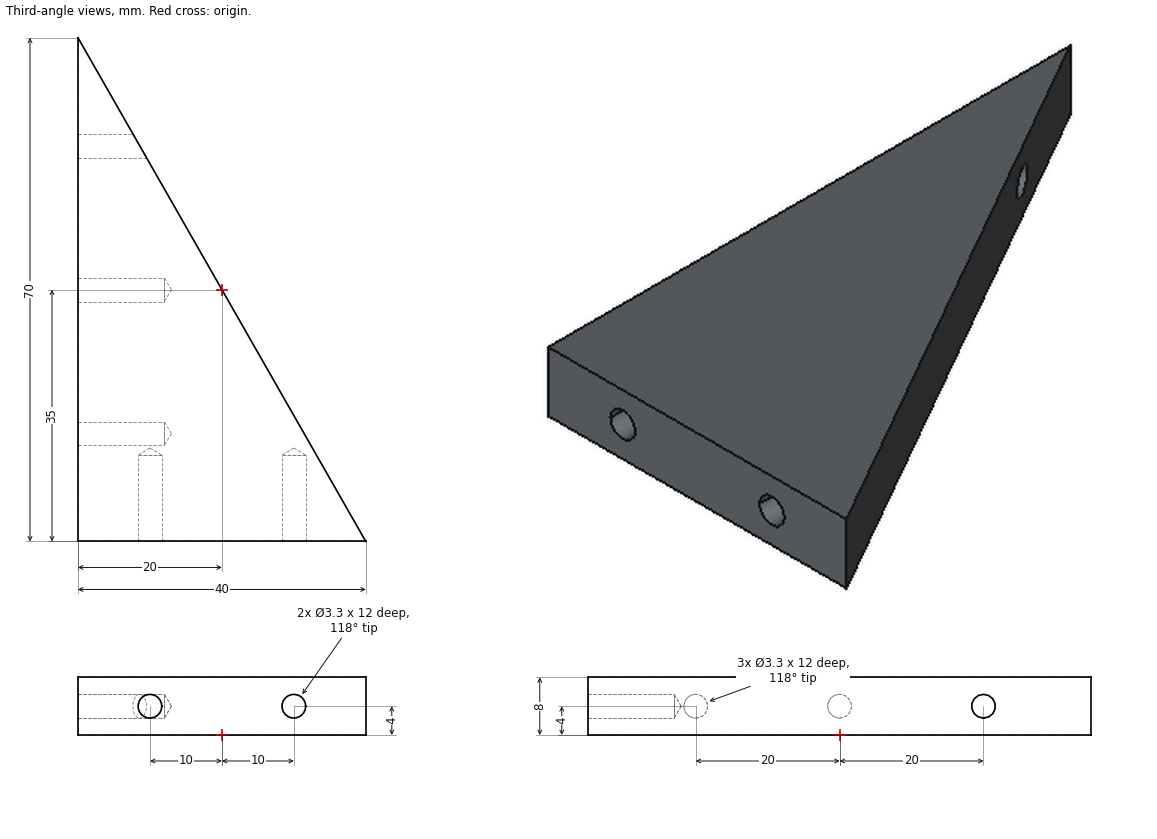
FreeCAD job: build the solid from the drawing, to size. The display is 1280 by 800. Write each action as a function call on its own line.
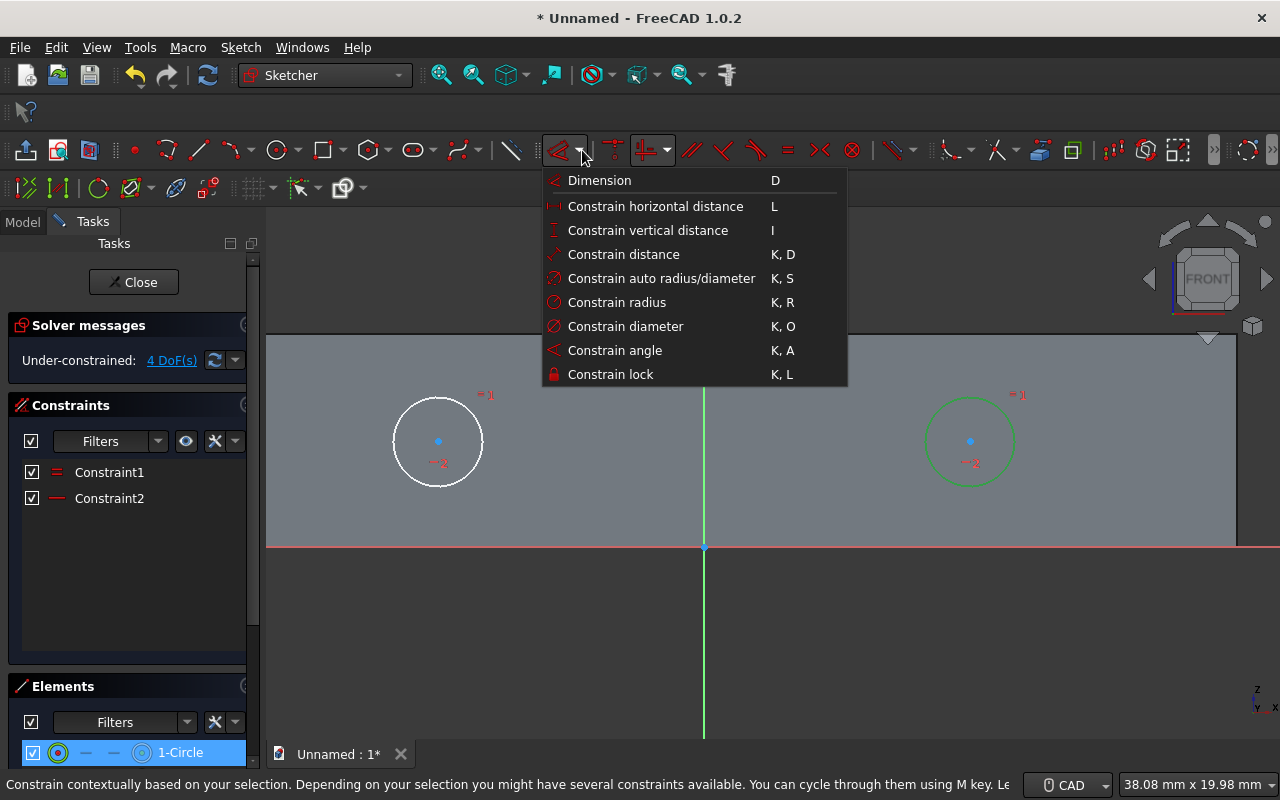
click(695, 326)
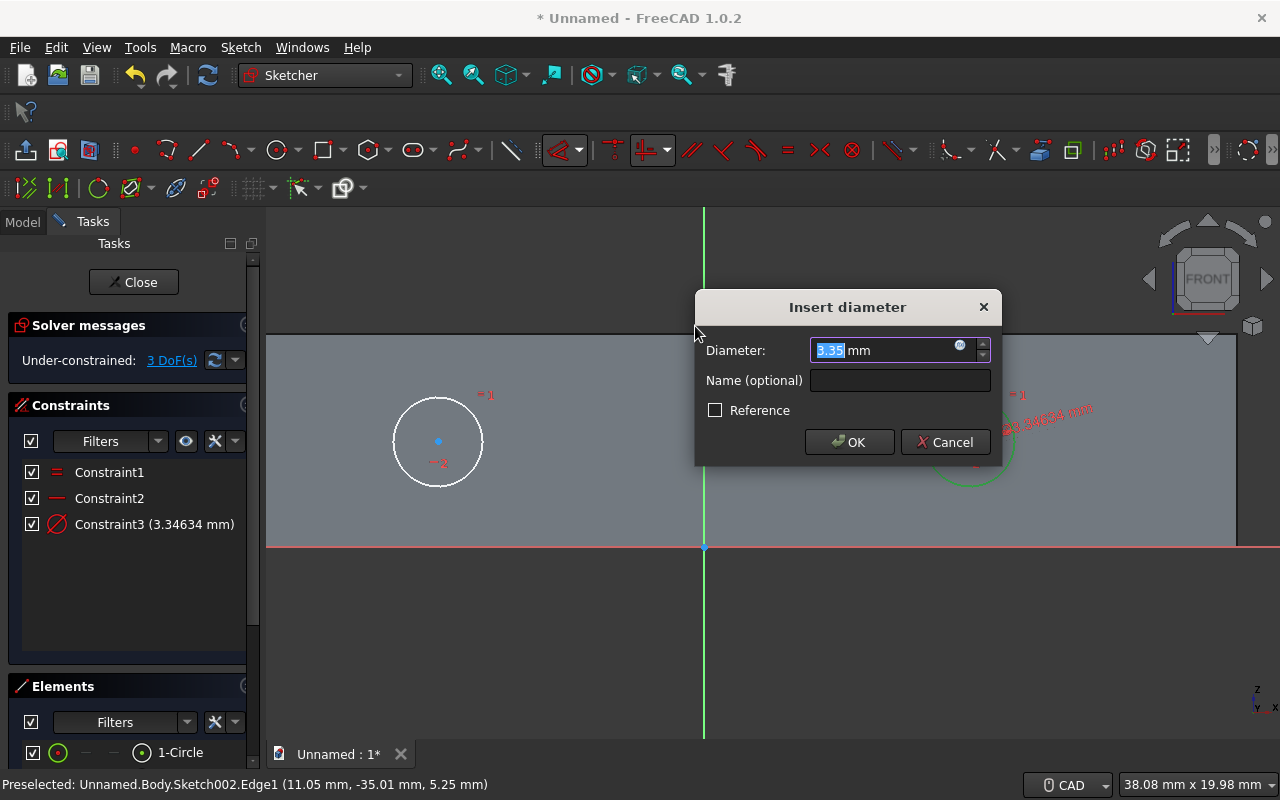
text(3.3)
key(Return)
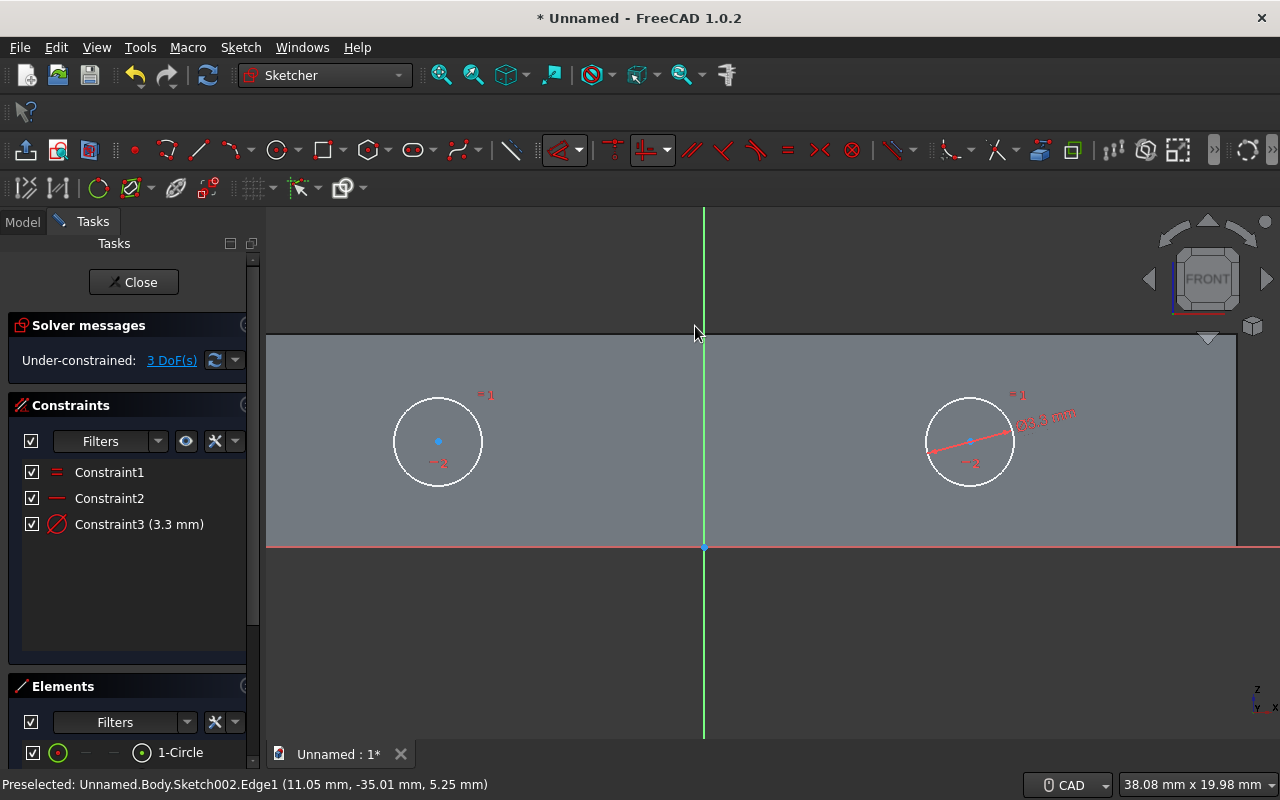
click(970, 442)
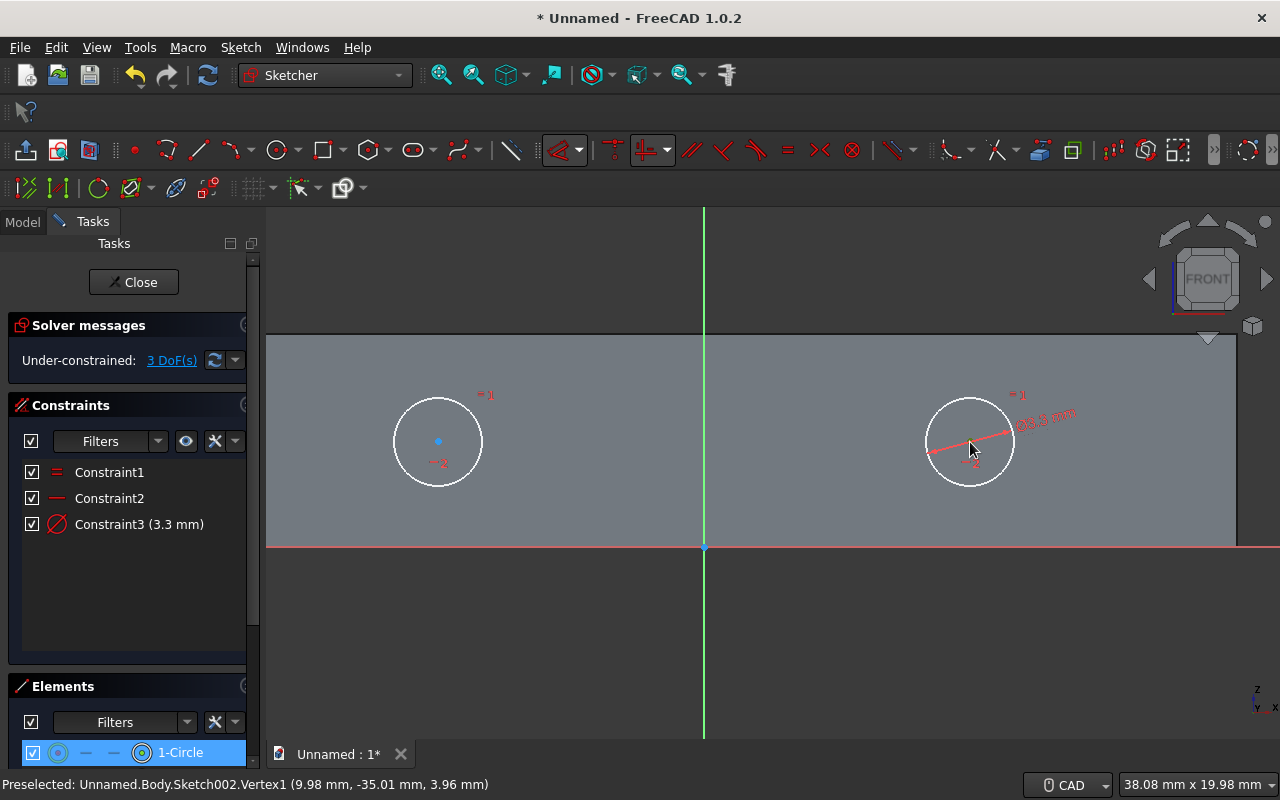
click(582, 150)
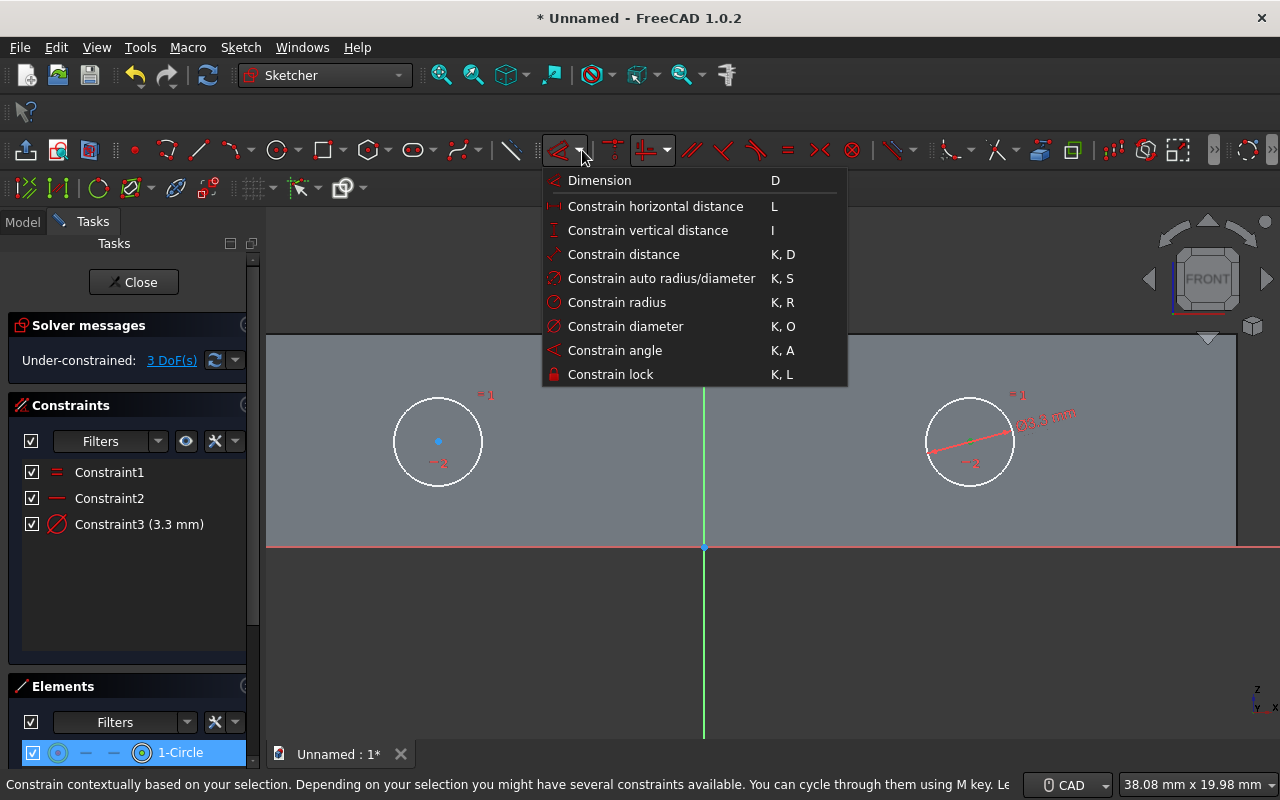
click(695, 230)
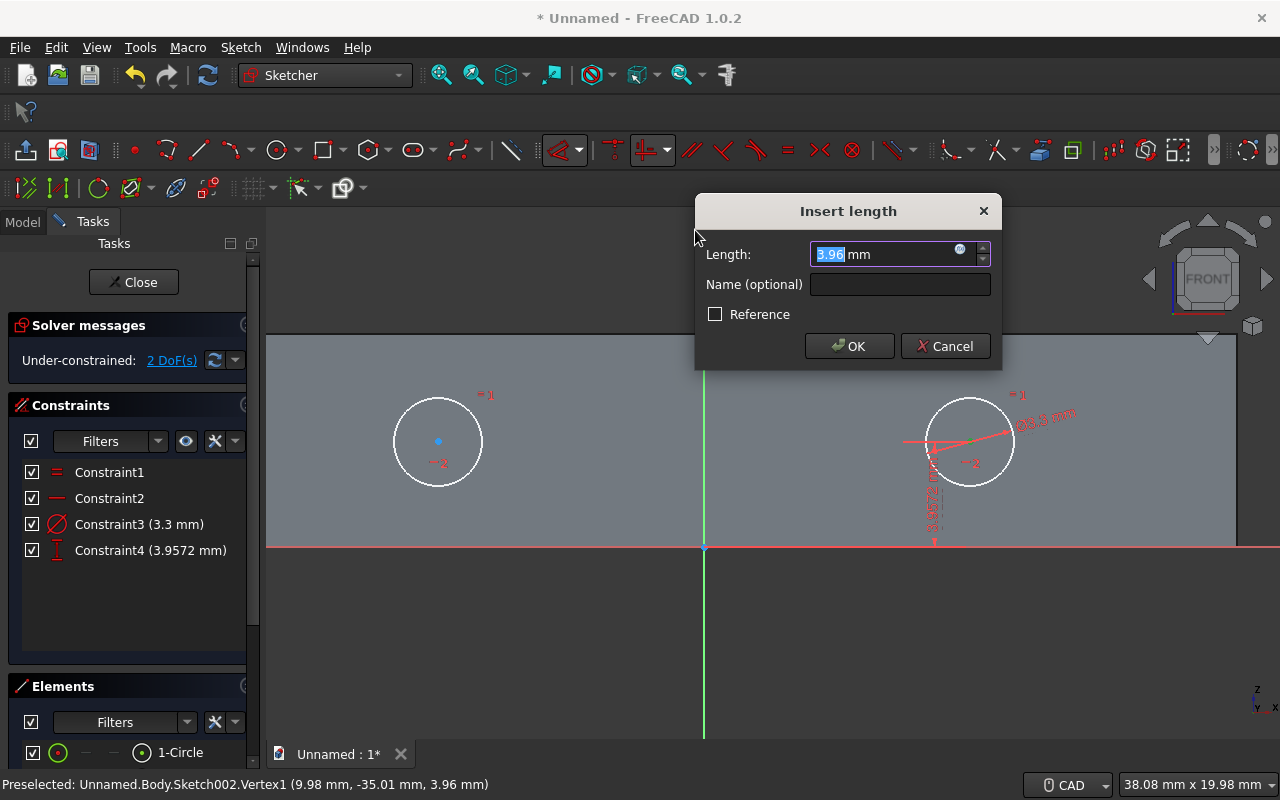
text(4)
key(Return)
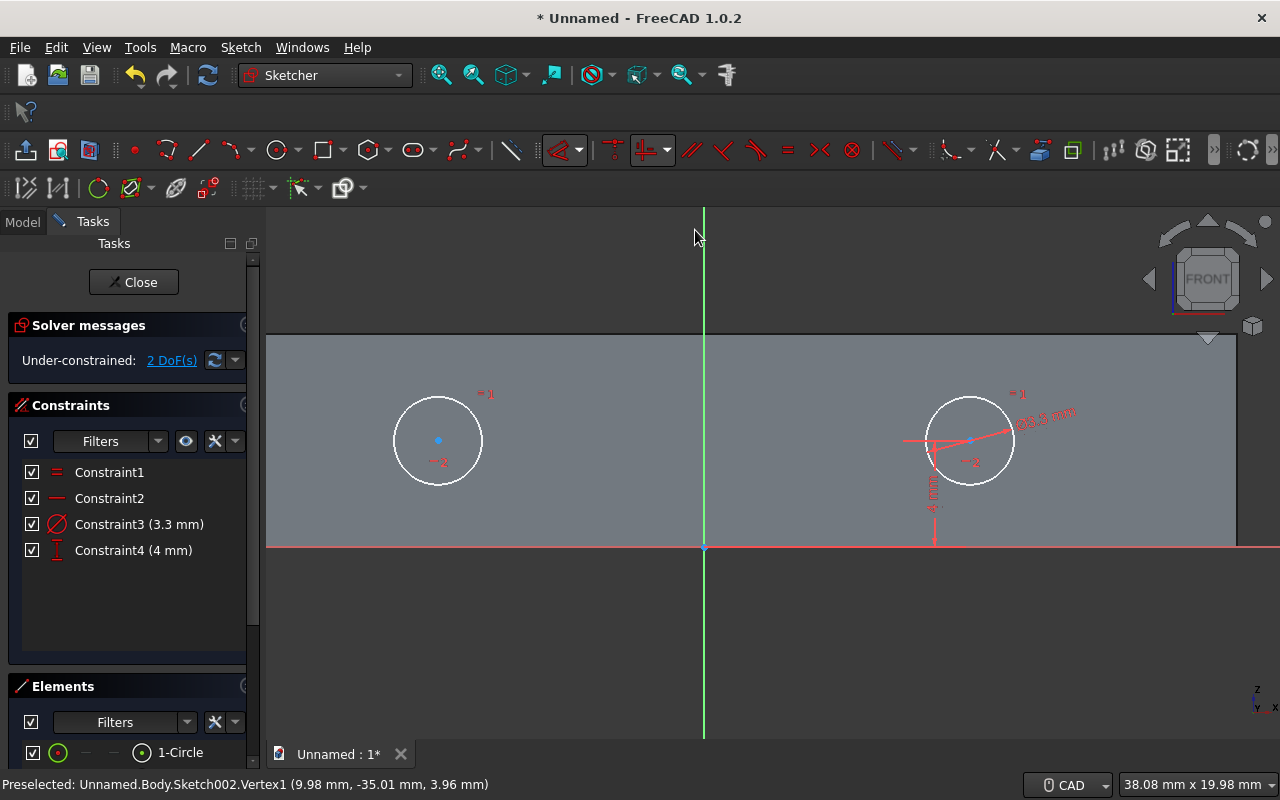
click(970, 441)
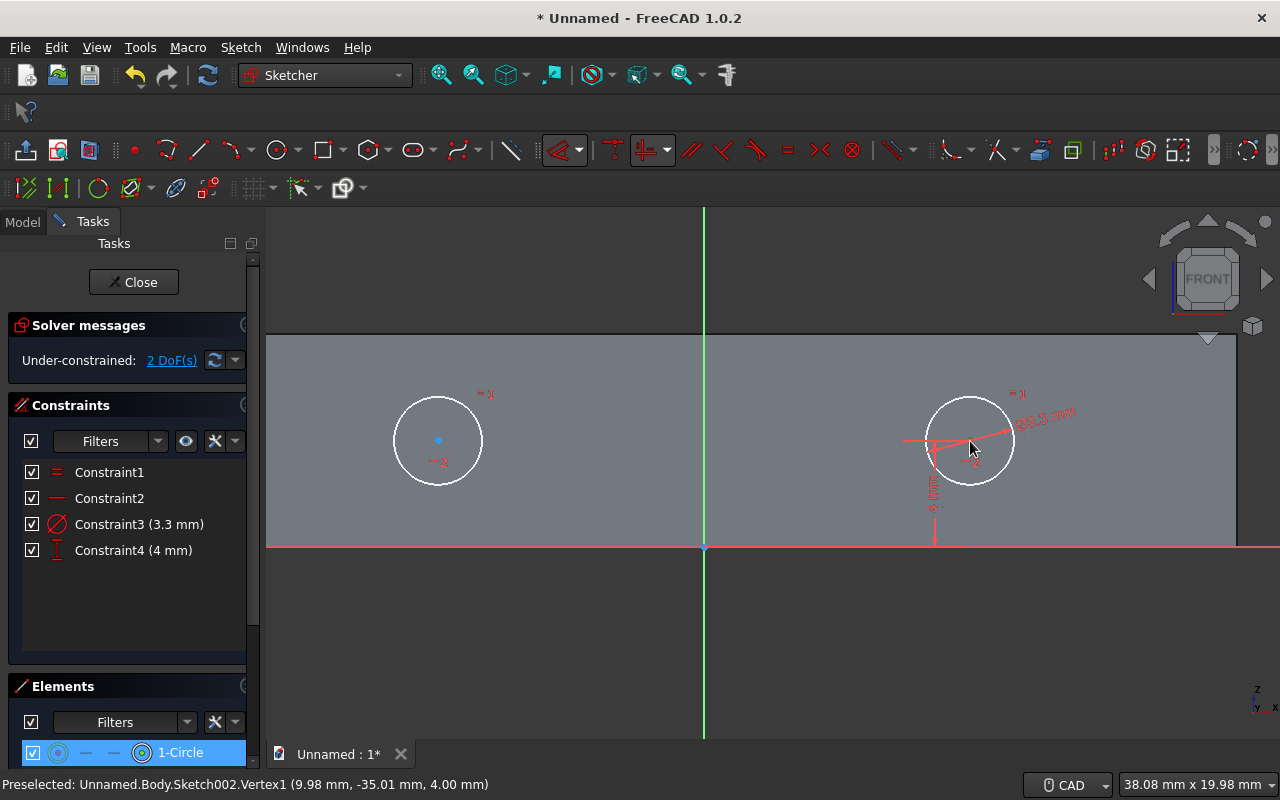
key(l)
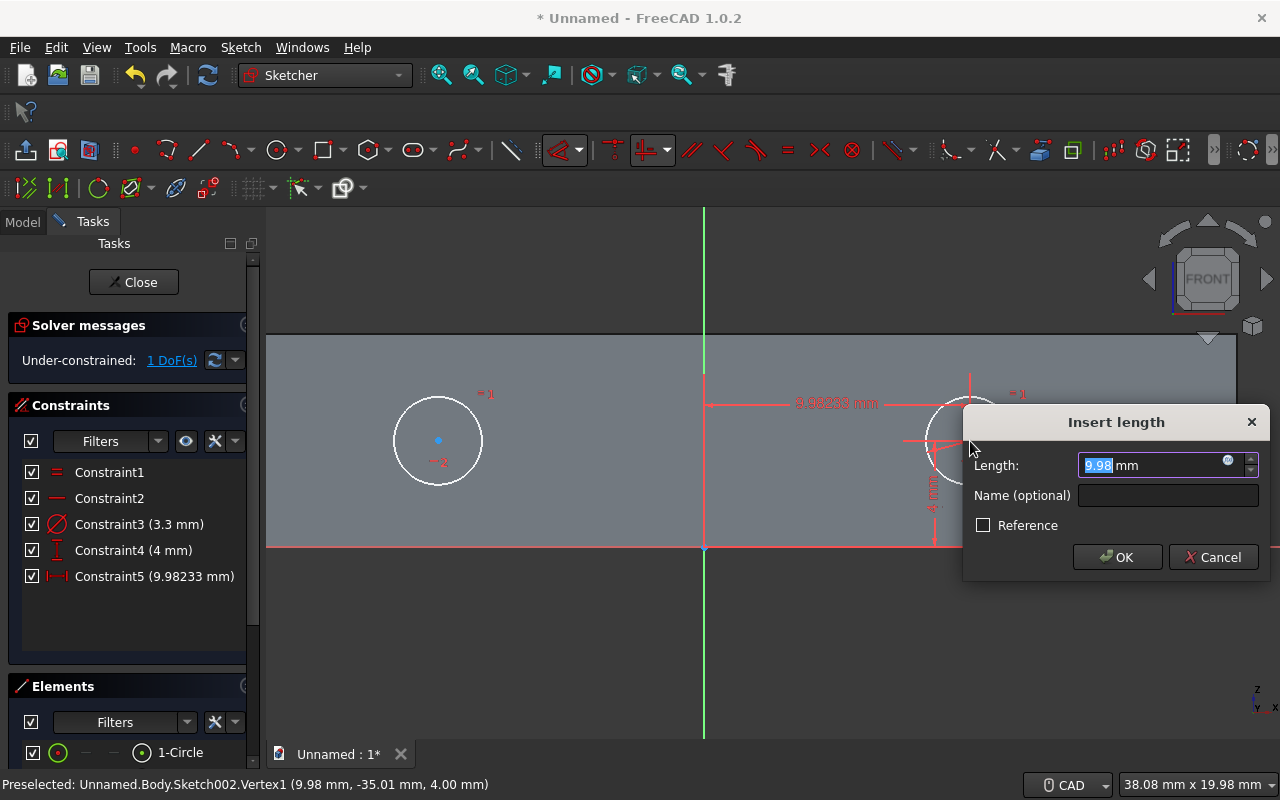
text(10)
key(Return)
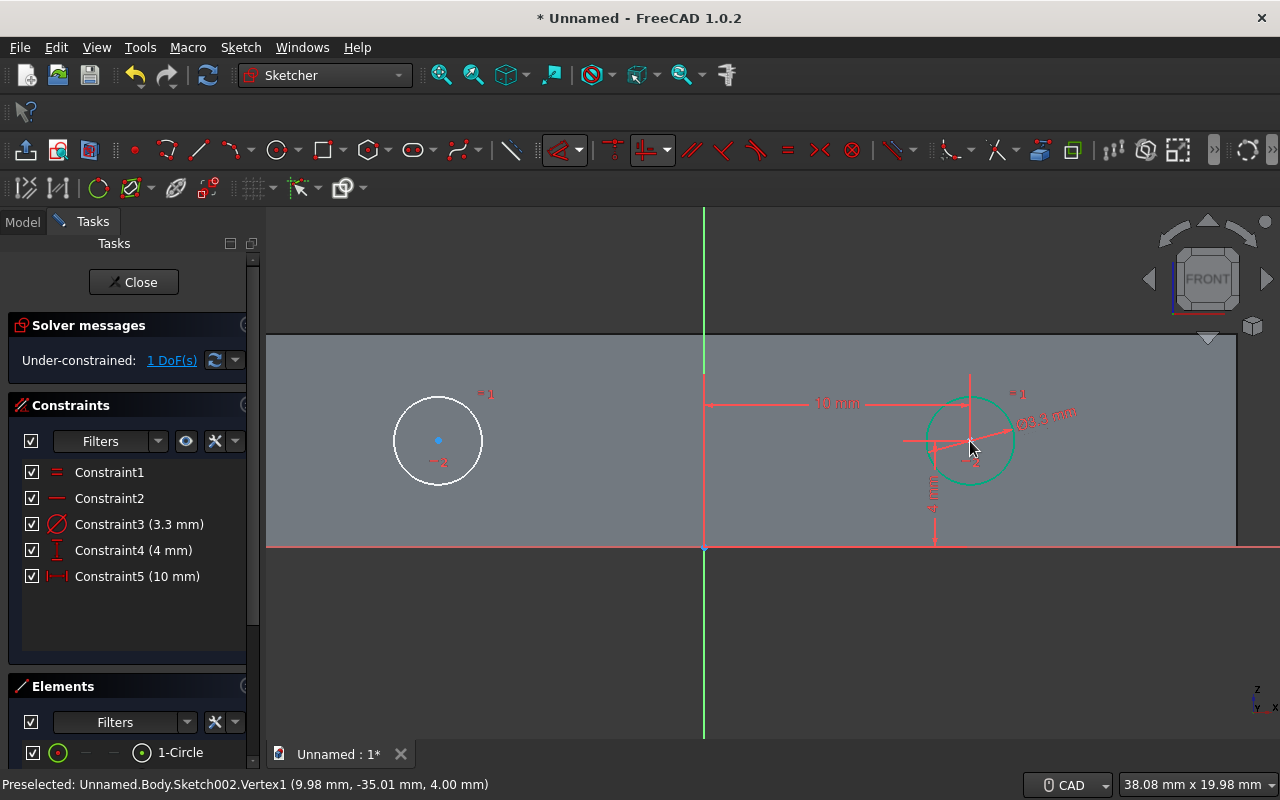
click(438, 441)